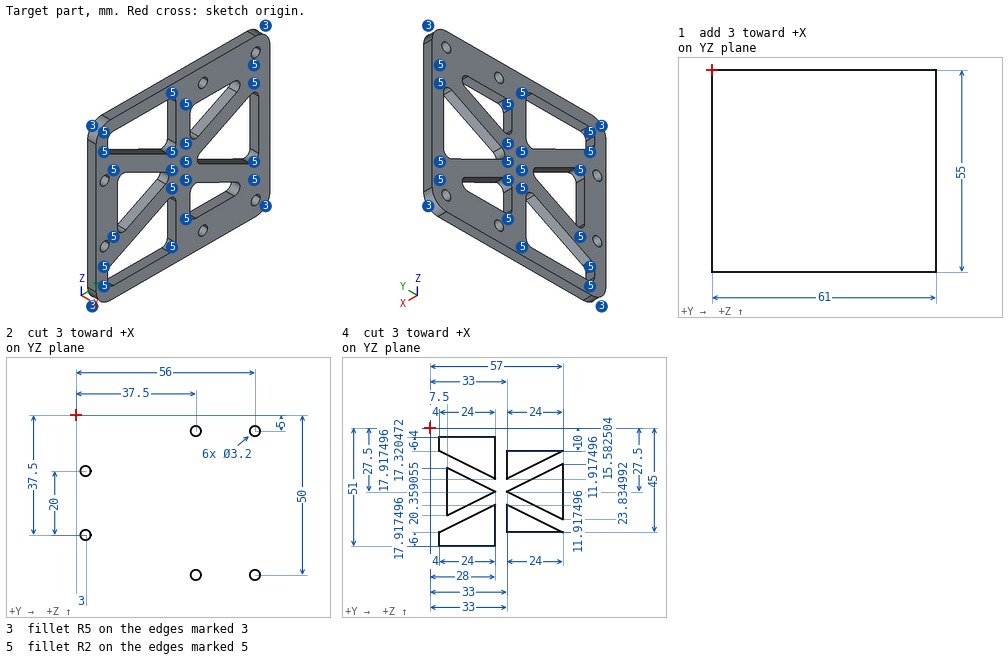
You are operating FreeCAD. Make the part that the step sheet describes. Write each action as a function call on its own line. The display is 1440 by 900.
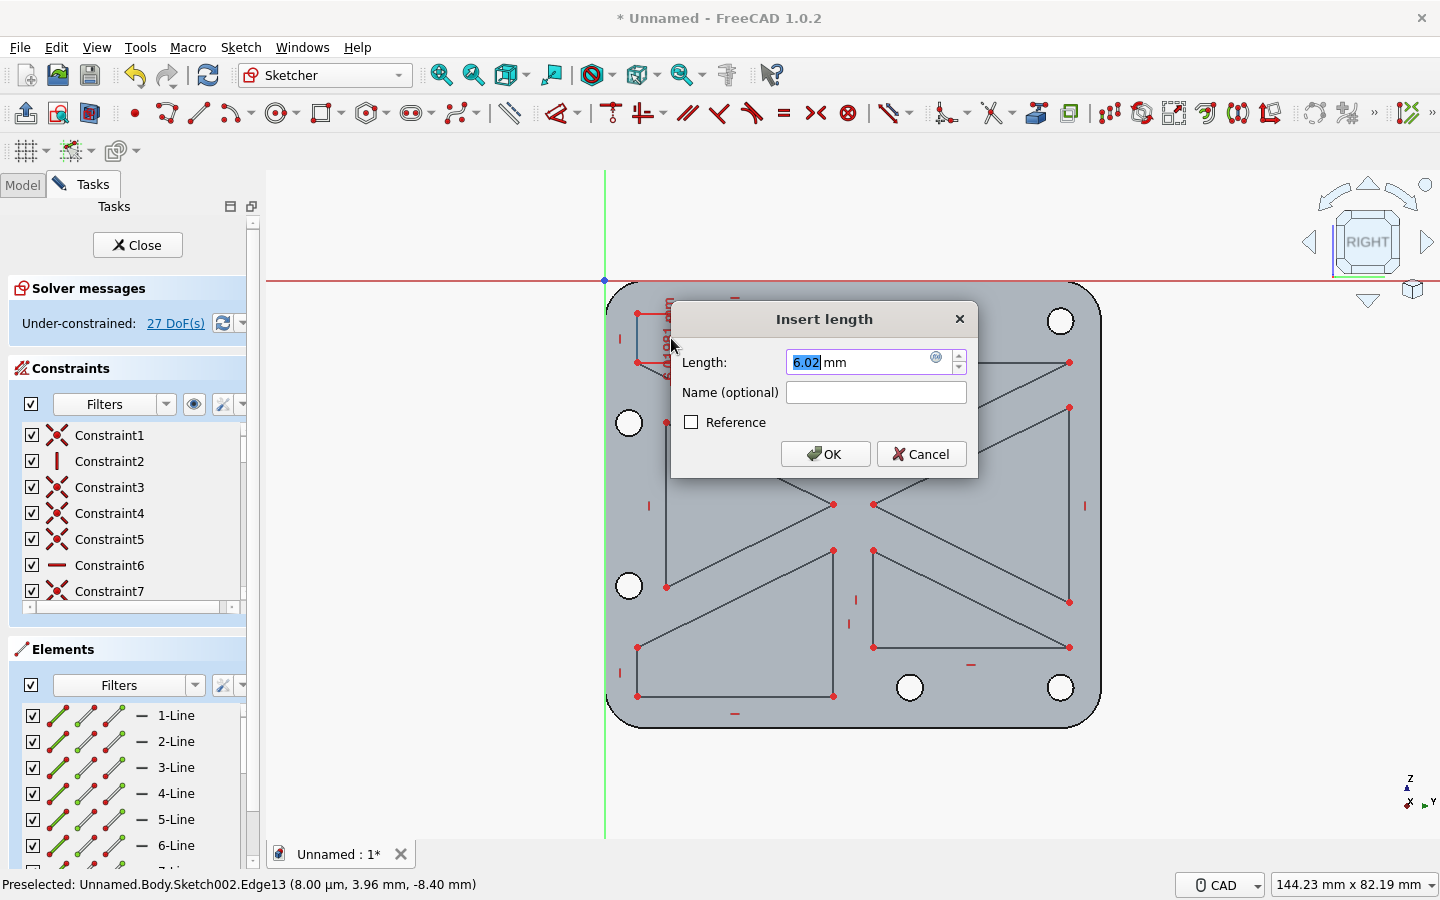
text(6)
key(Return)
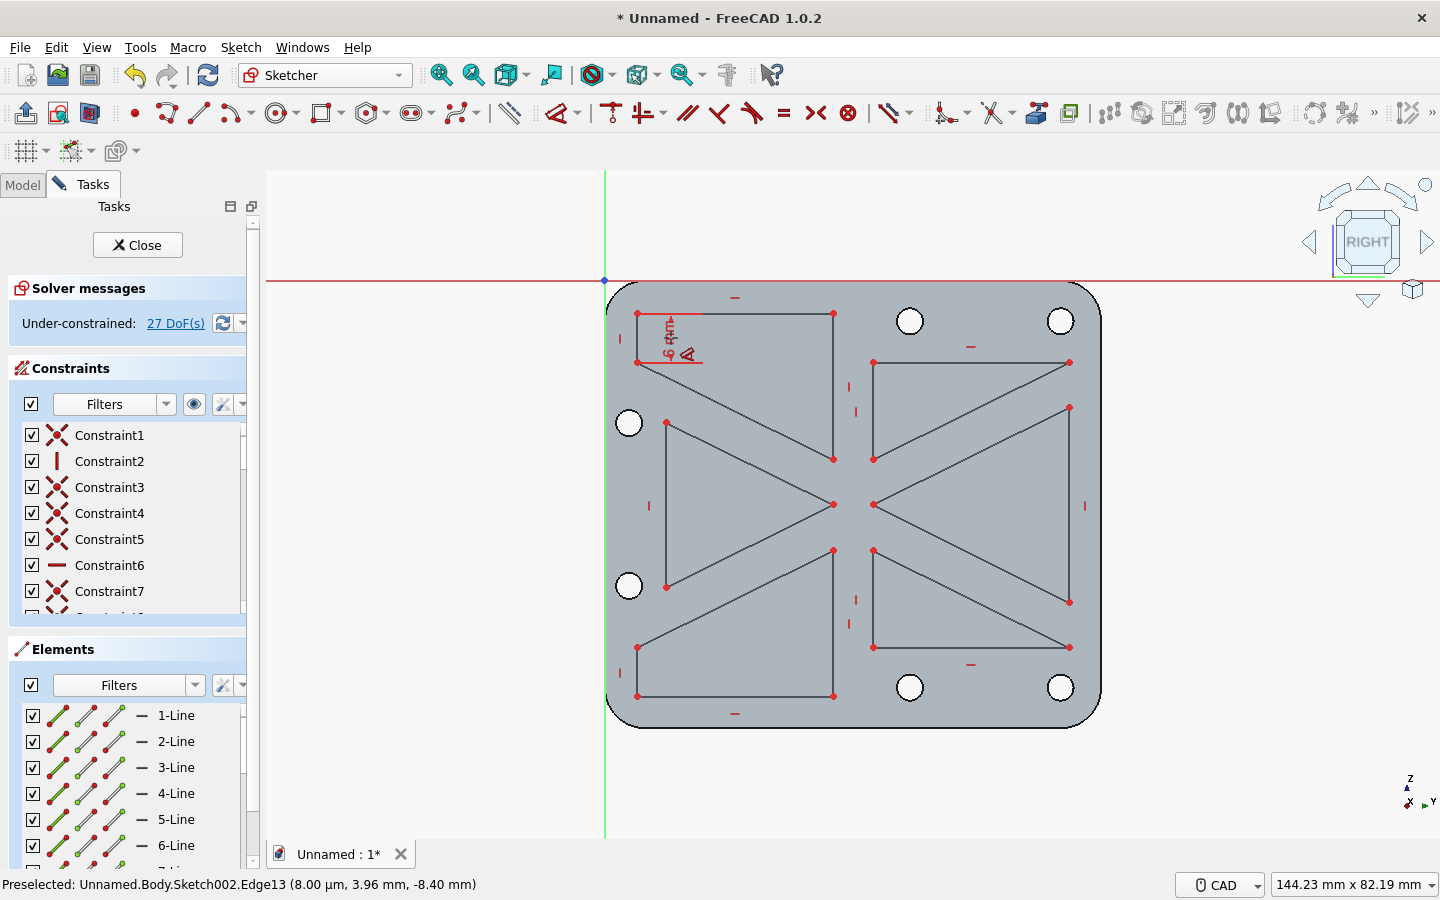
click(637, 682)
click(671, 673)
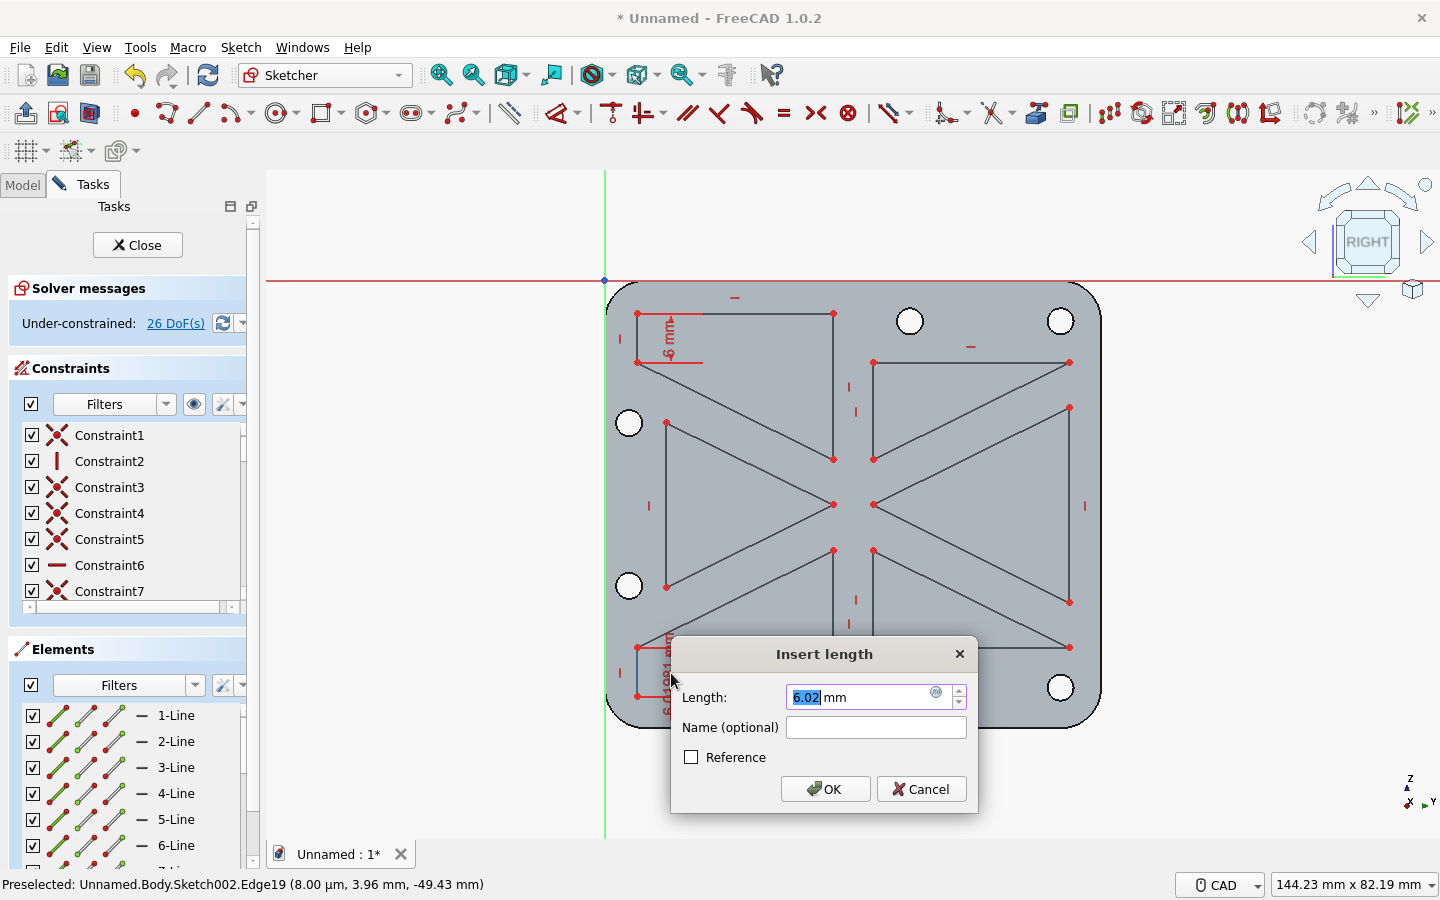
text(6)
key(Return)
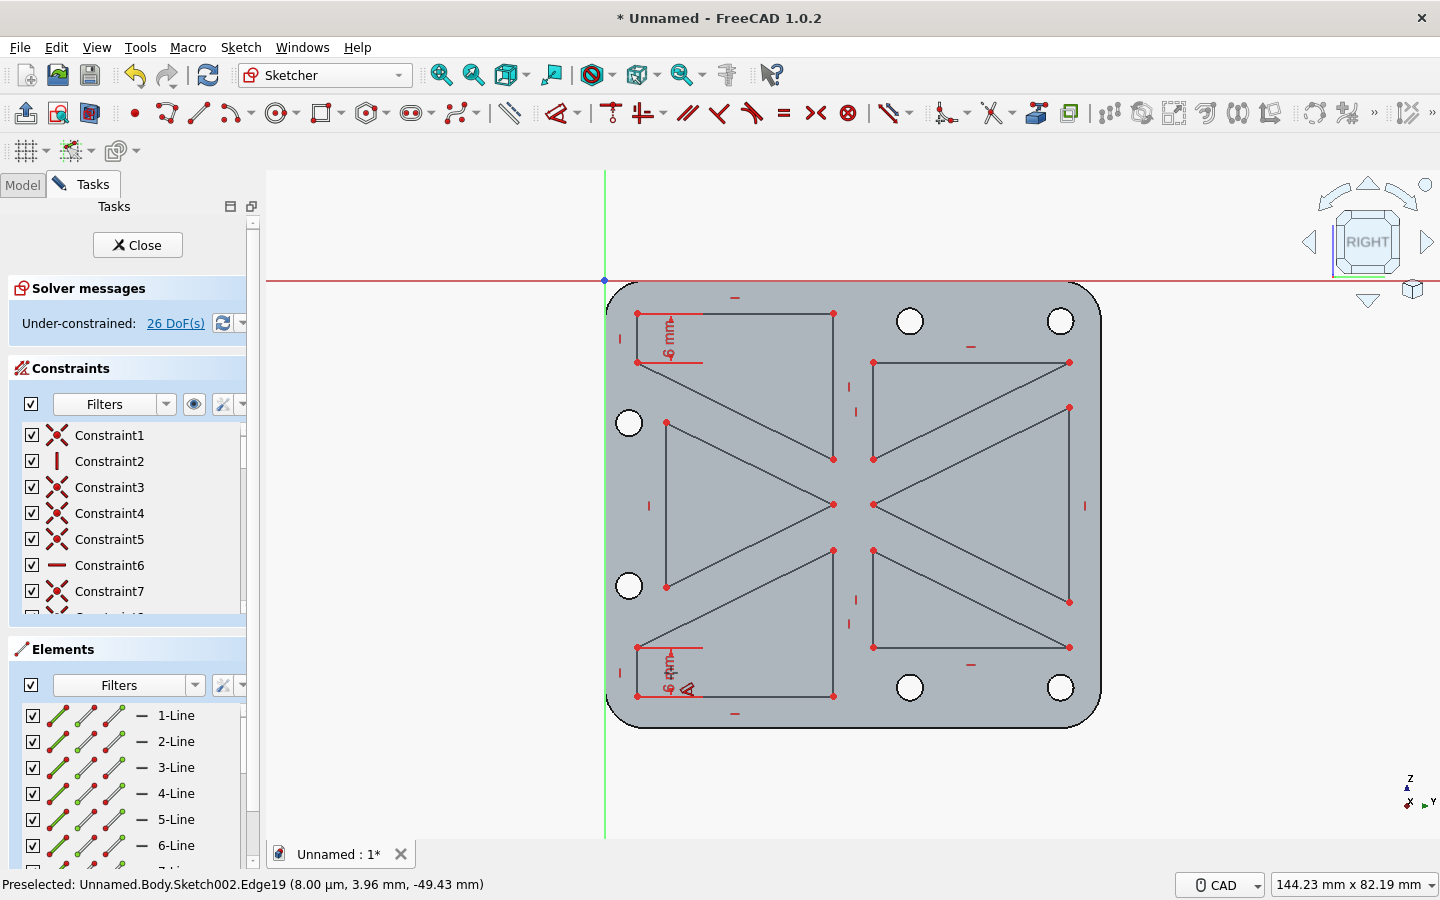
click(1010, 648)
click(971, 682)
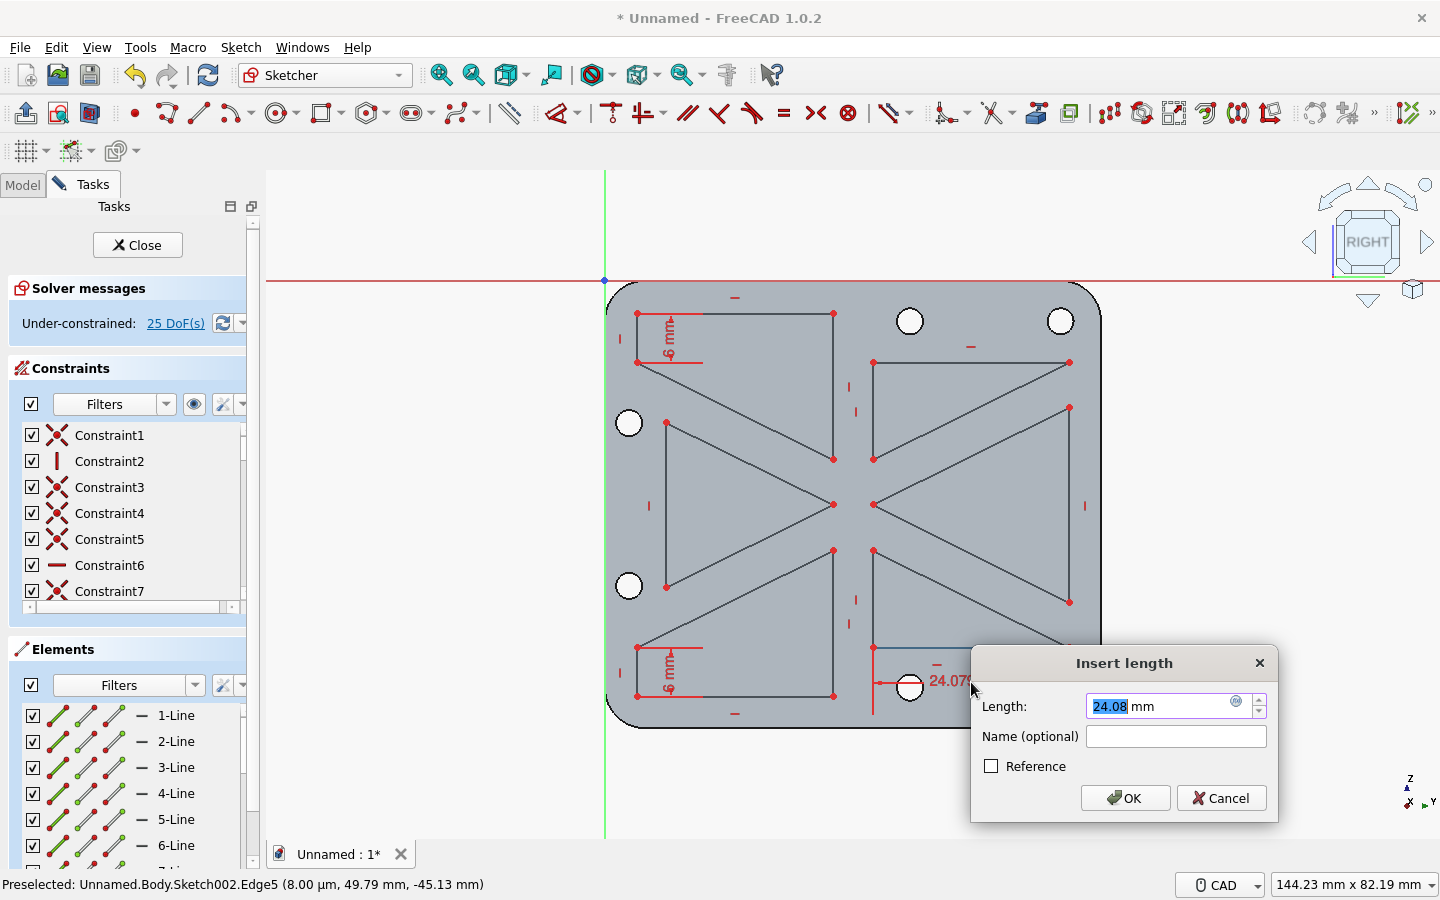
text(24)
key(Return)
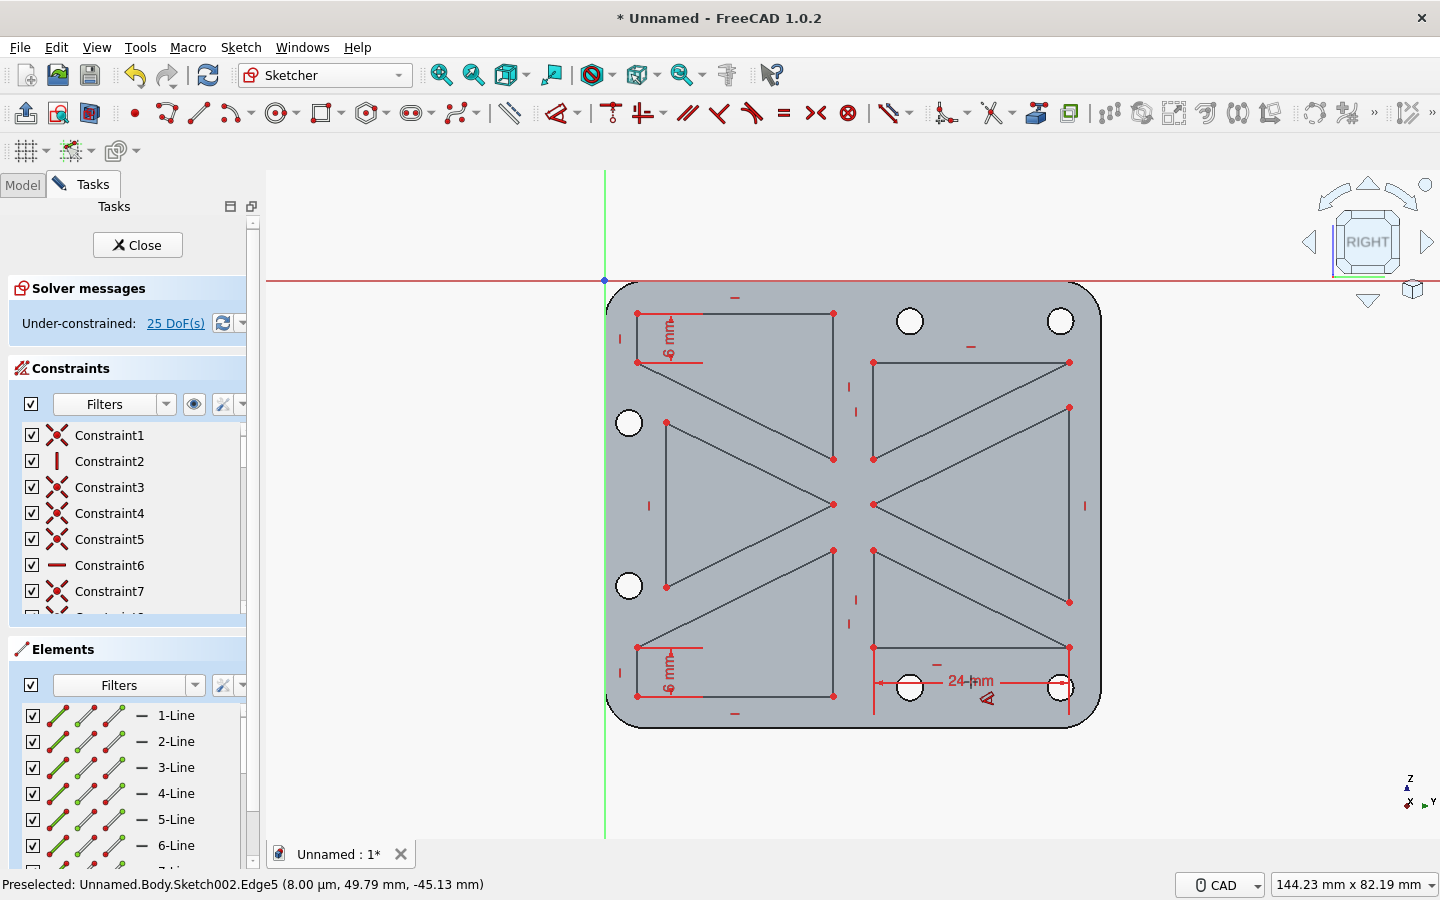
click(932, 363)
click(971, 329)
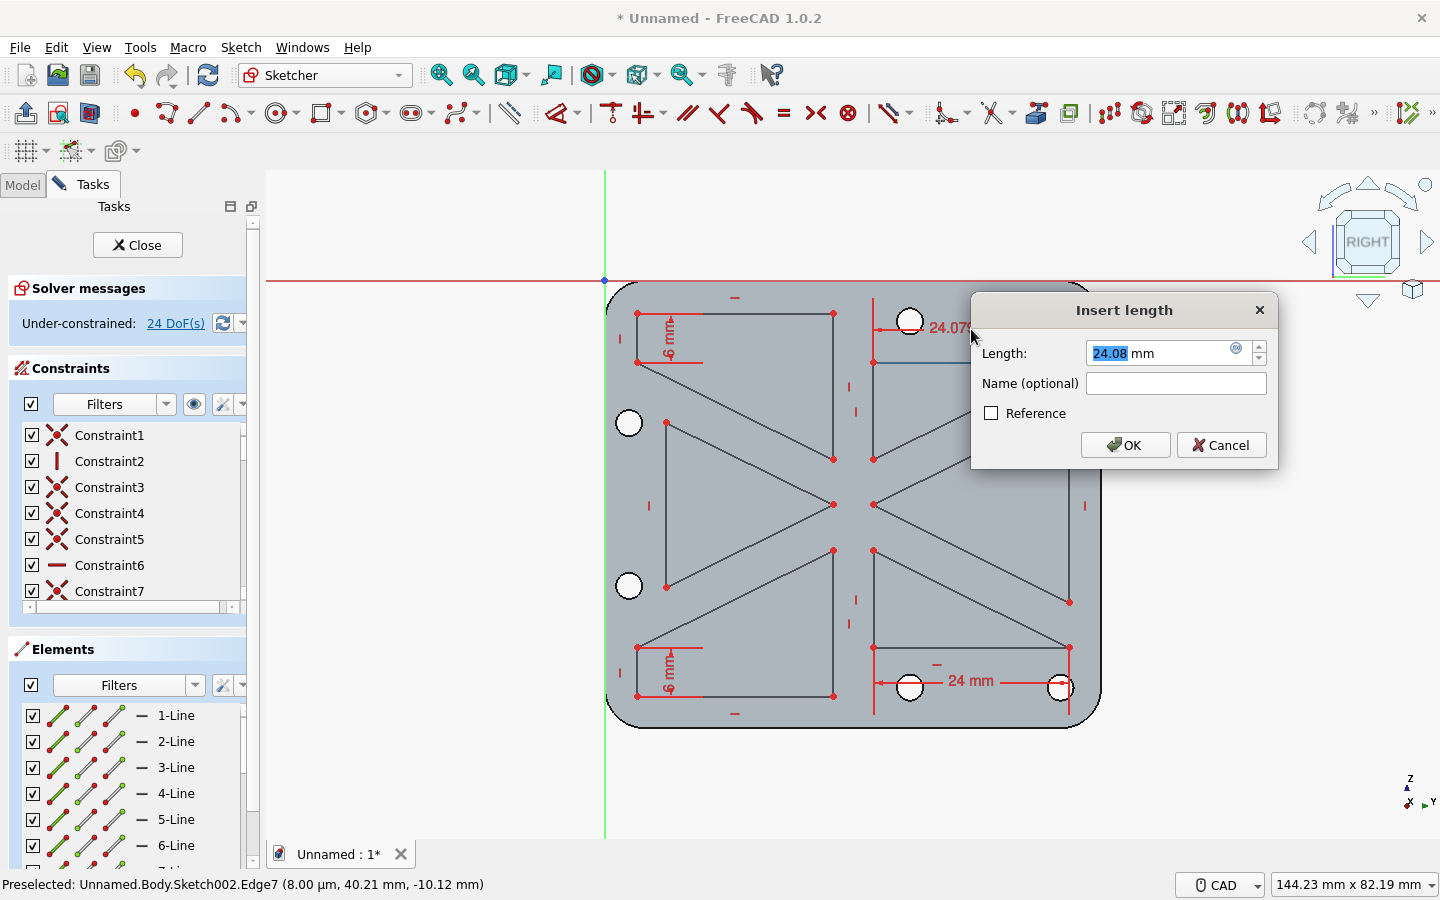
text(24)
key(Return)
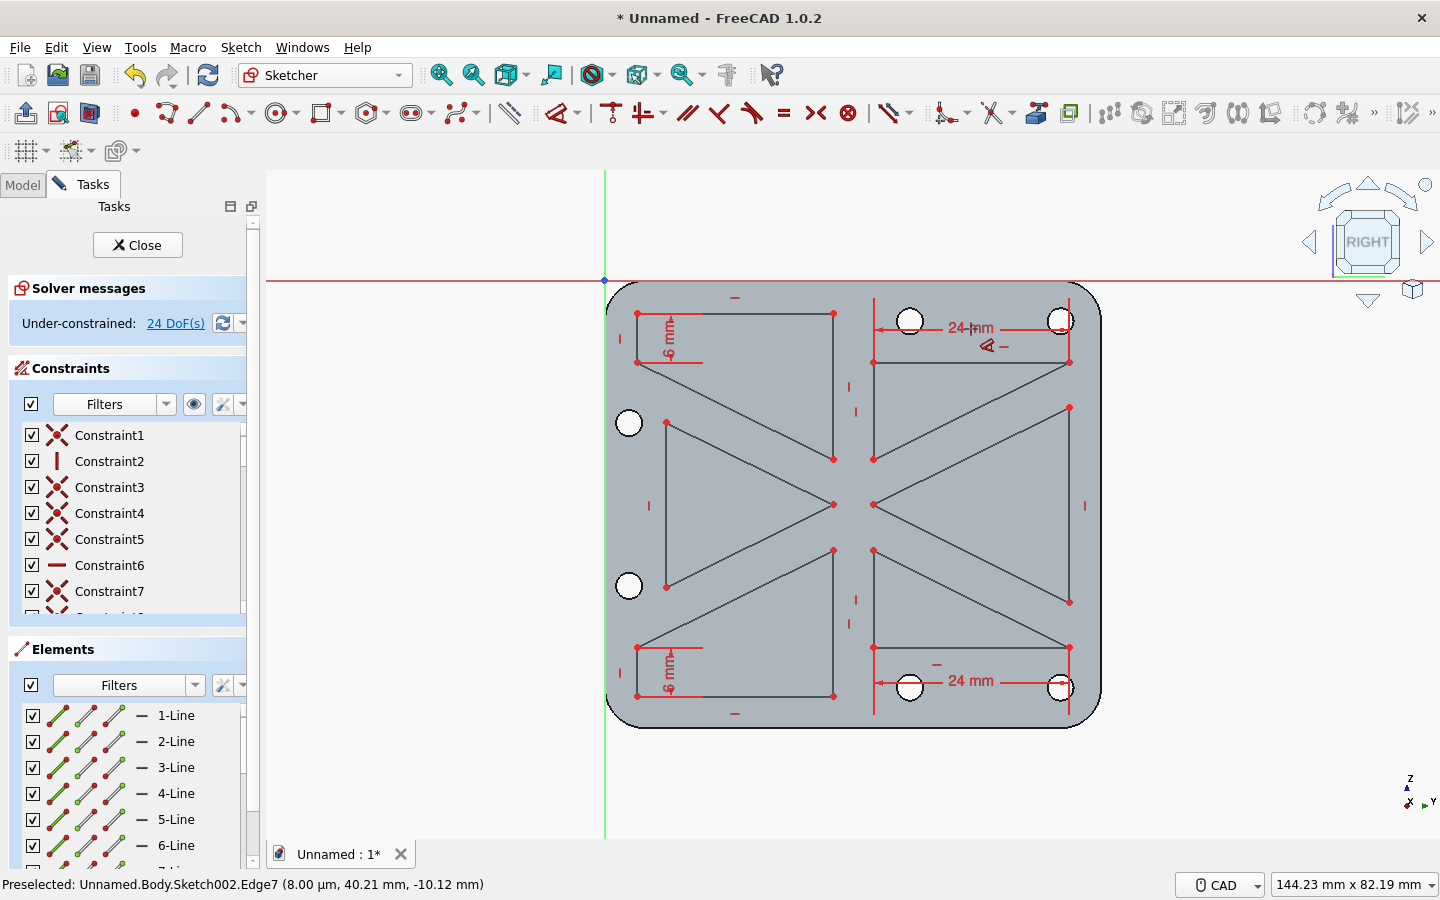
click(696, 314)
click(780, 348)